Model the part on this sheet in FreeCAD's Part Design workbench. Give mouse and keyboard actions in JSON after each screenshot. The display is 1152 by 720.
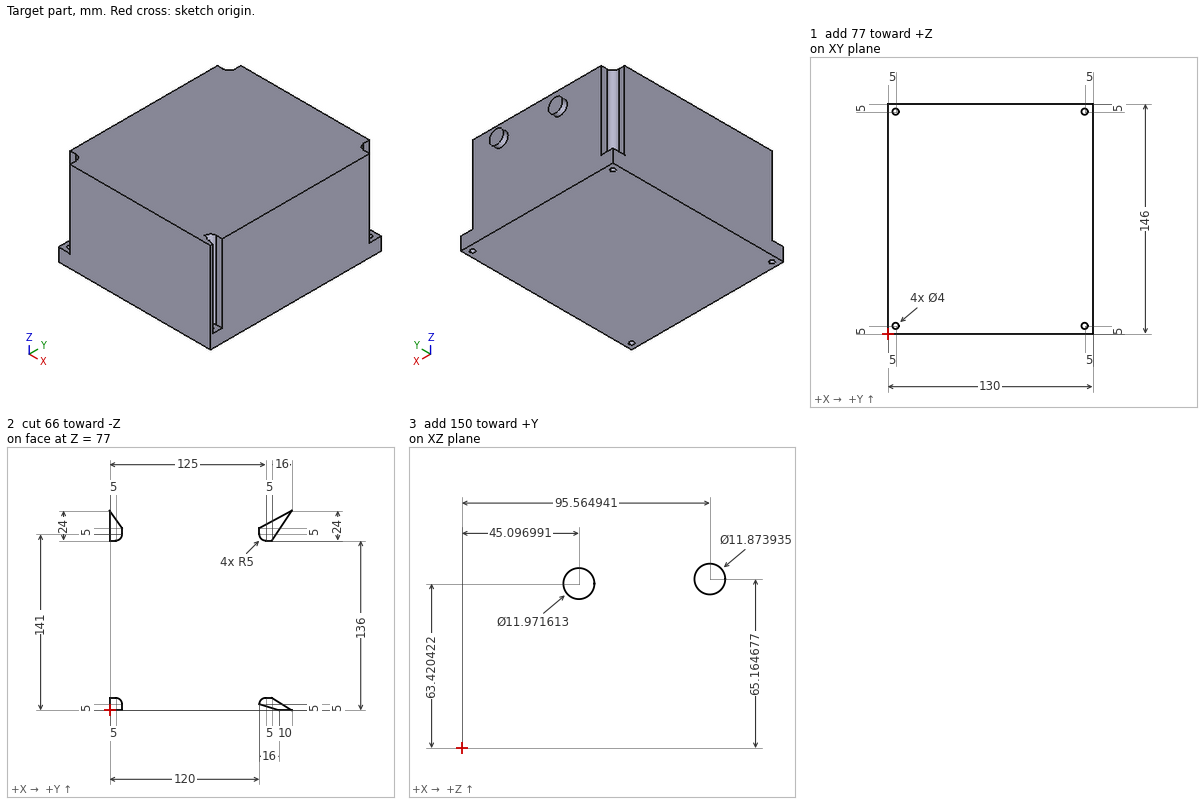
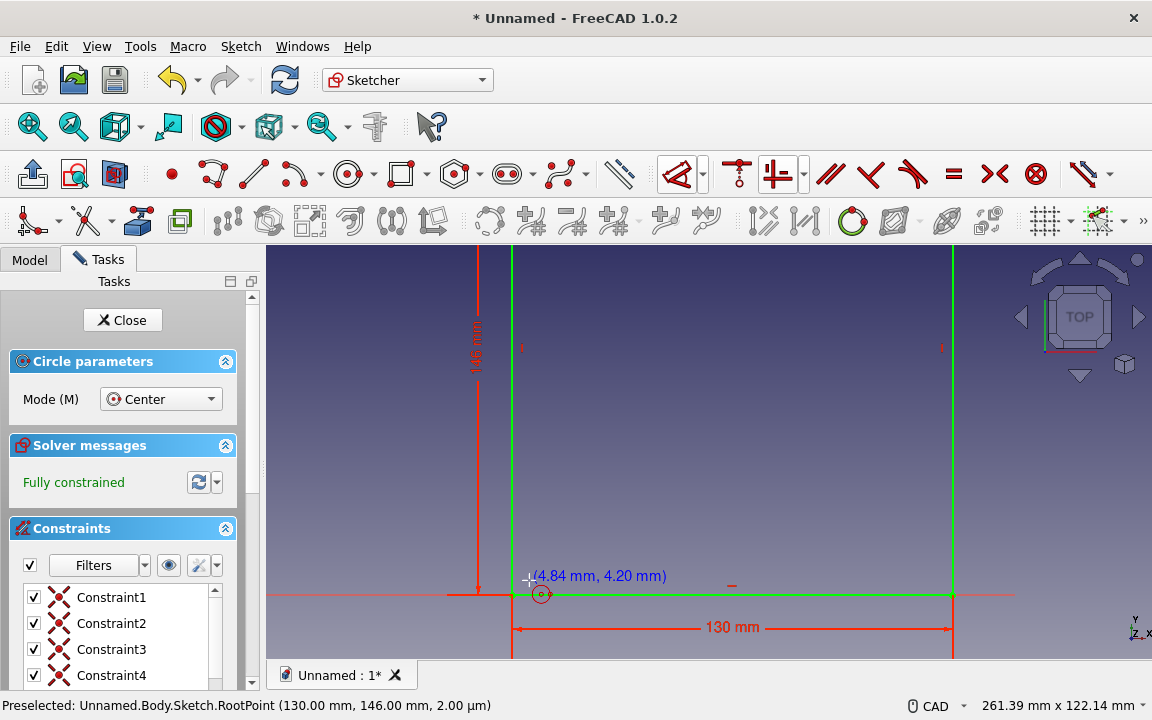
{"action": "left_click", "coordinate": [529, 578]}
{"action": "mouse_move", "coordinate": [534, 574]}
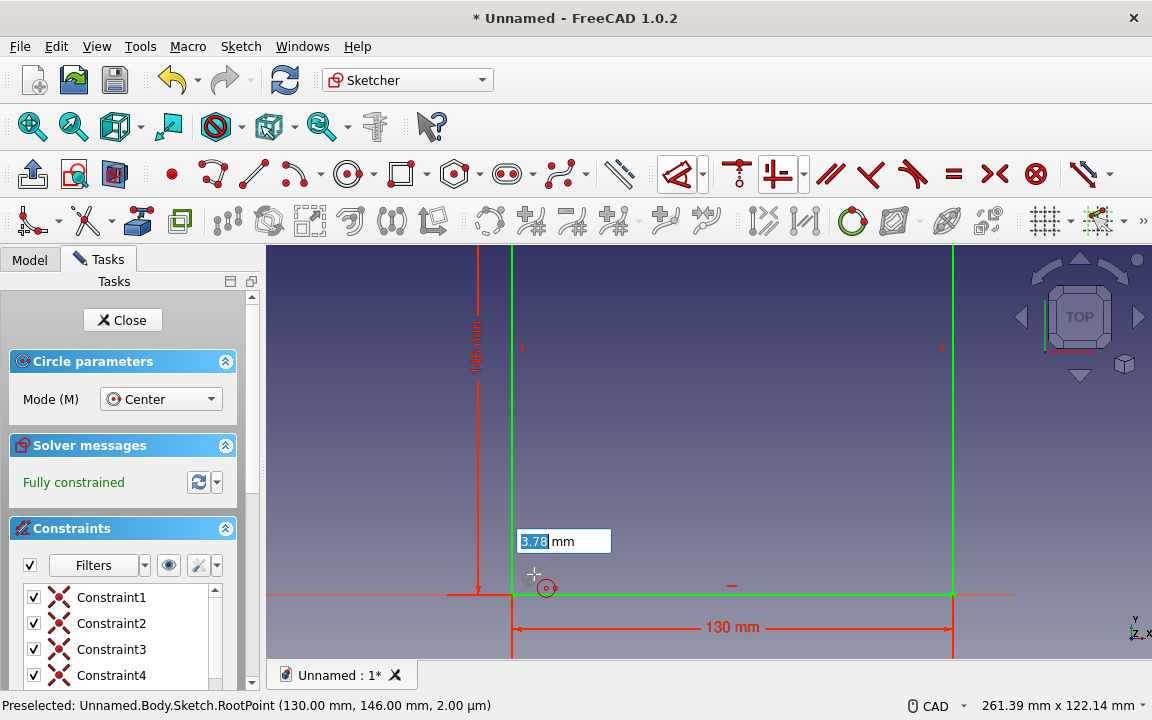
{"action": "type", "text": "4"}
{"action": "key", "text": "Return"}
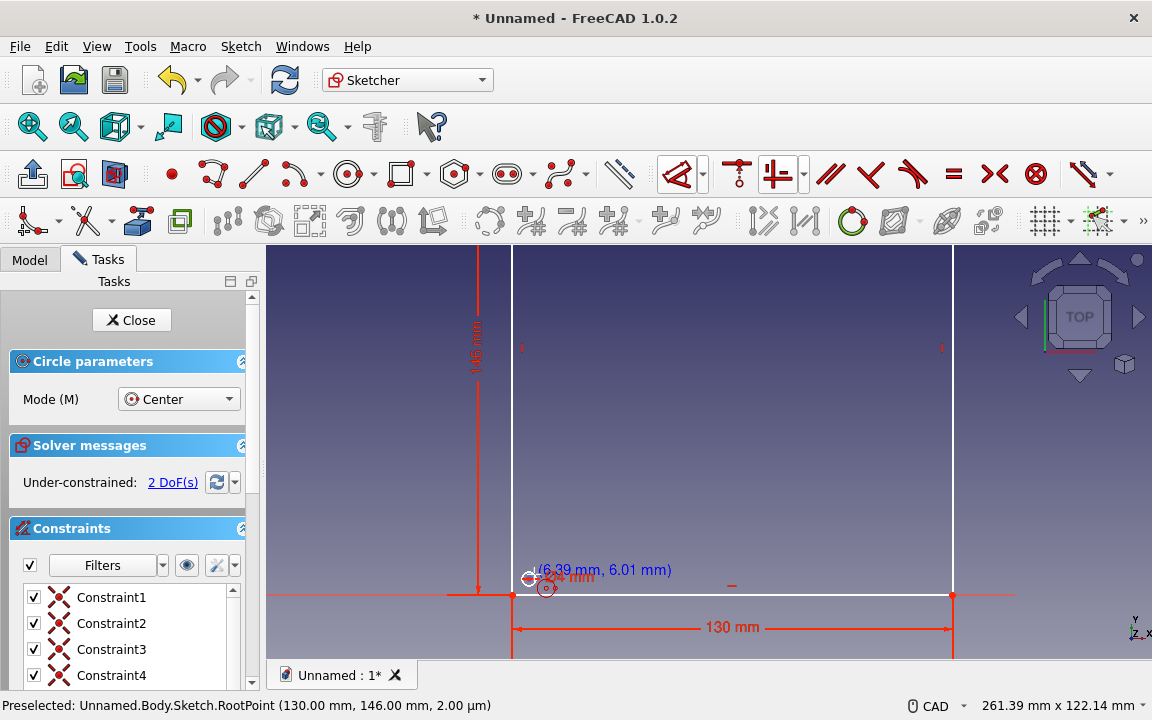
{"action": "scroll", "coordinate": [936, 578], "scroll_direction": "up", "scroll_amount": 7}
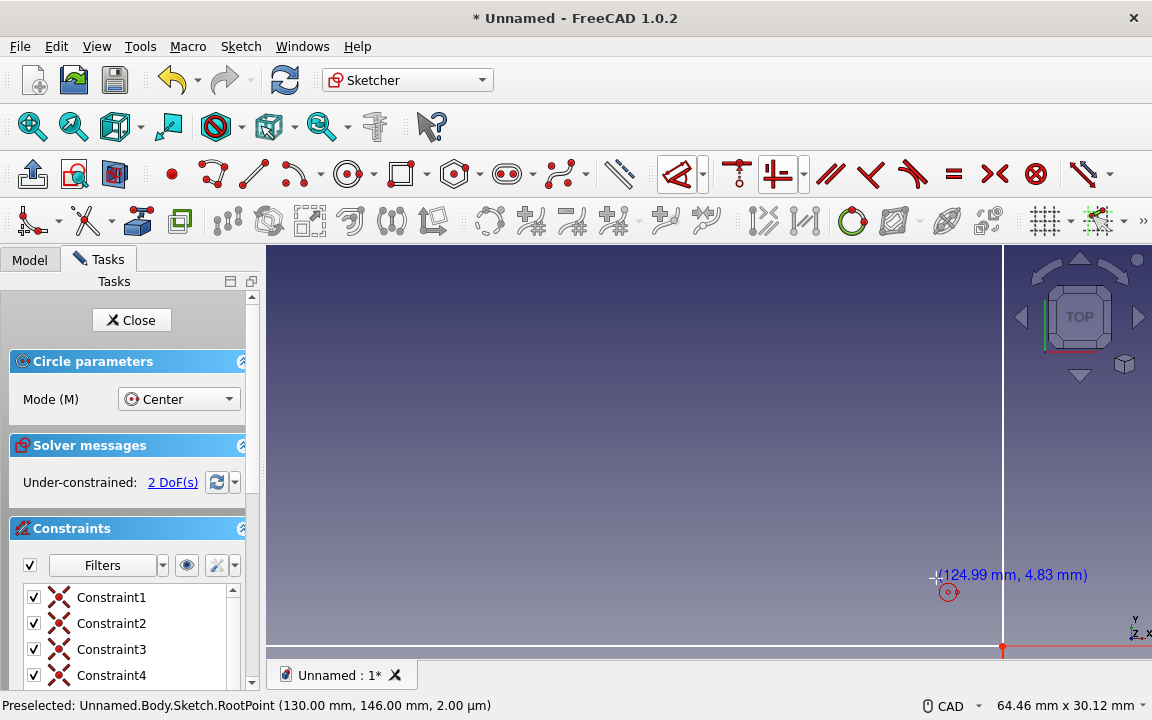
{"action": "scroll", "coordinate": [724, 579], "scroll_direction": "down", "scroll_amount": 10}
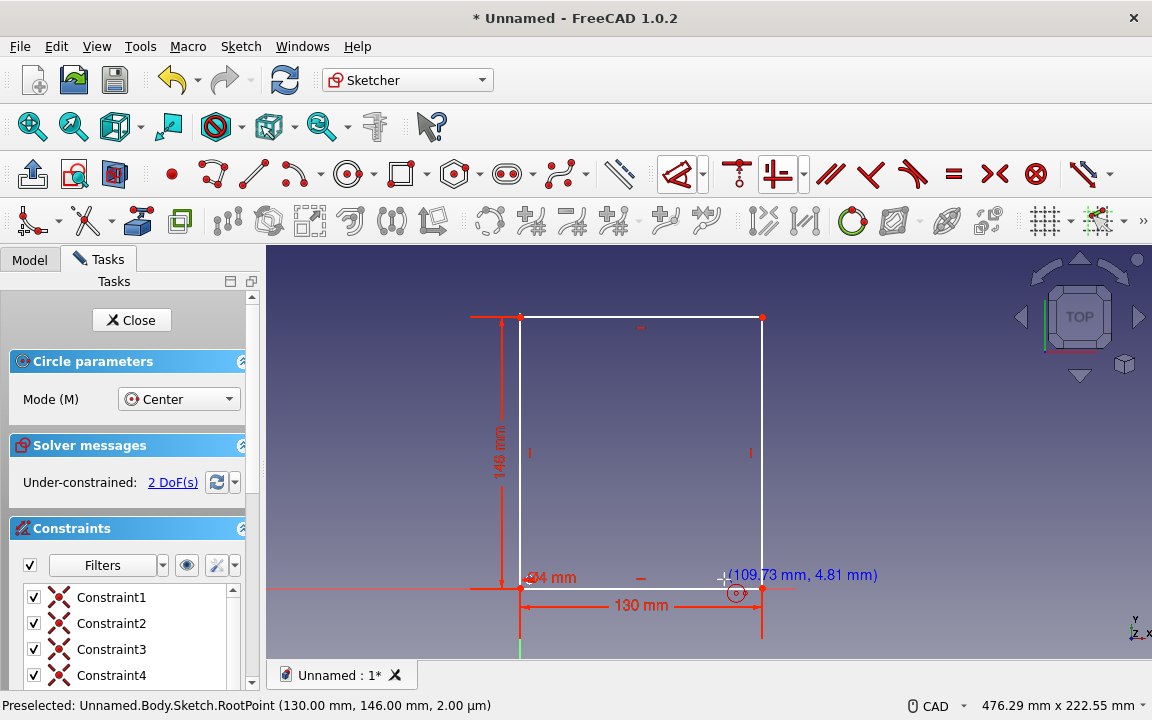
{"action": "scroll", "coordinate": [753, 579], "scroll_direction": "up", "scroll_amount": 3}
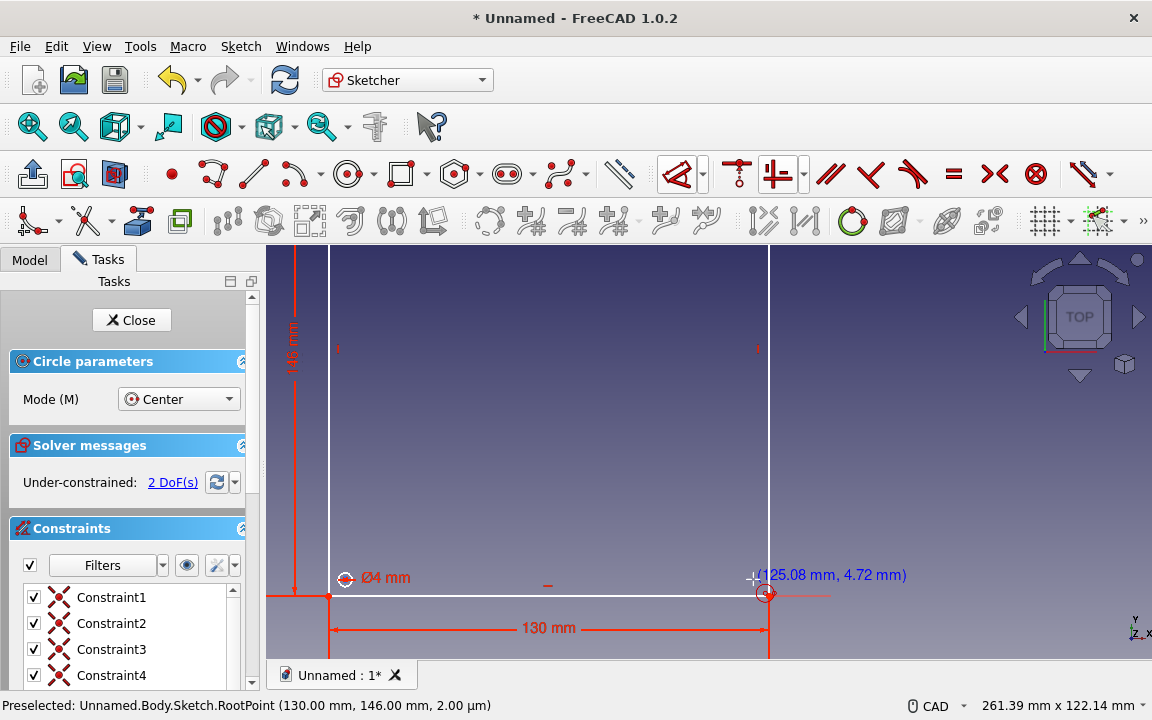
{"action": "left_click", "coordinate": [752, 579]}
{"action": "mouse_move", "coordinate": [747, 574]}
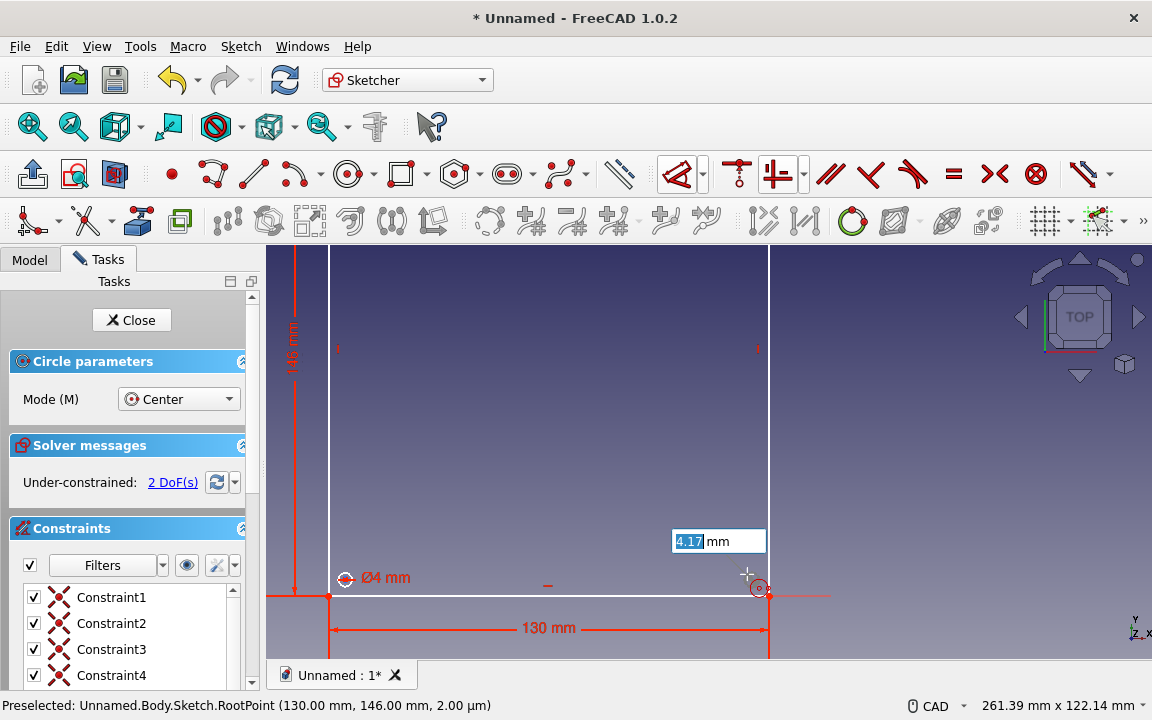
{"action": "type", "text": "4"}
{"action": "key", "text": "Return"}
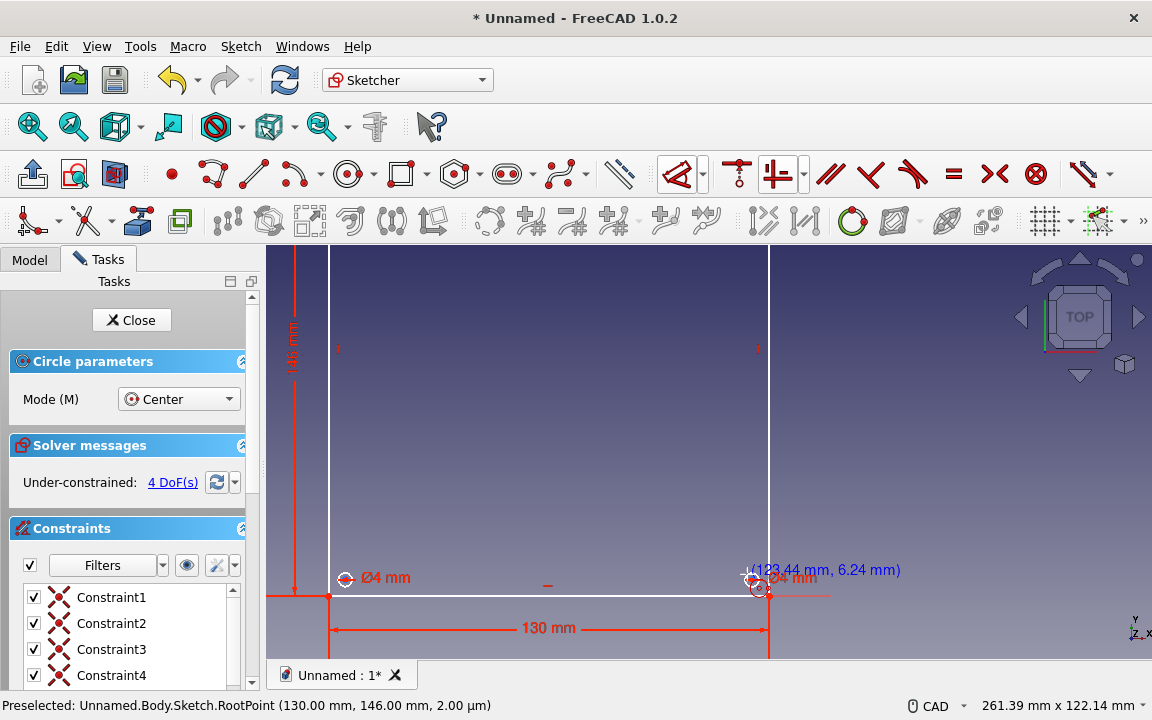
{"action": "scroll", "coordinate": [752, 578], "scroll_direction": "down", "scroll_amount": 3}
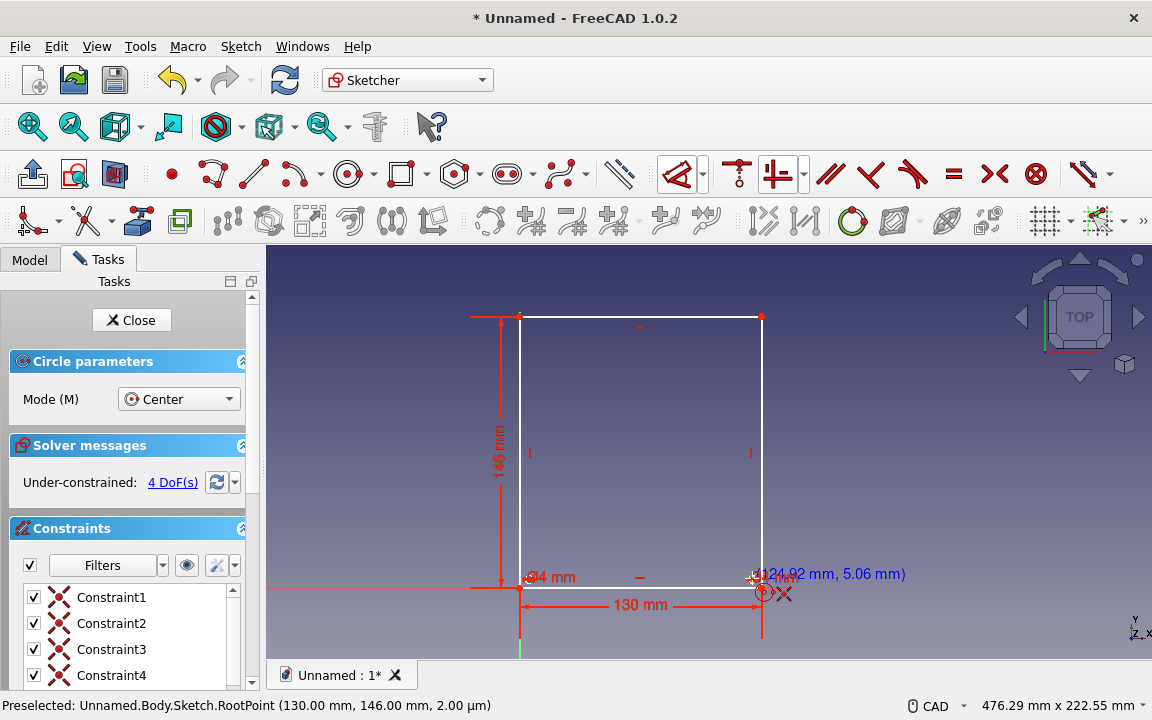
{"action": "scroll", "coordinate": [529, 326], "scroll_direction": "up", "scroll_amount": 10}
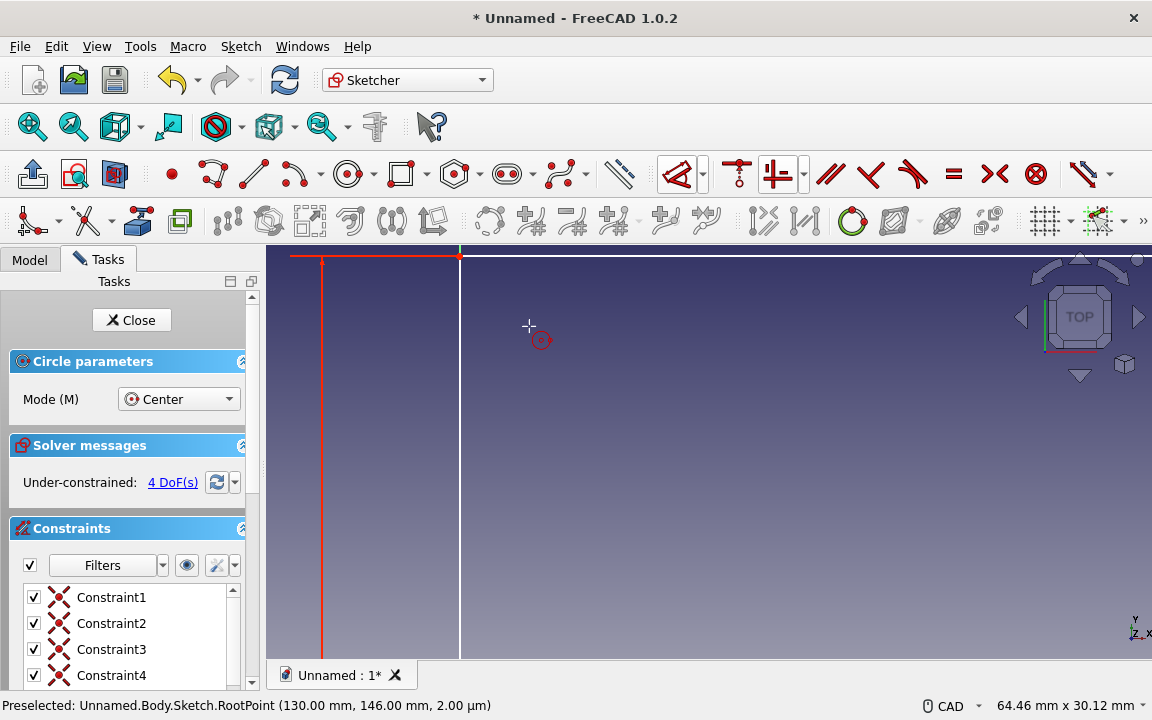
{"action": "scroll", "coordinate": [529, 326], "scroll_direction": "down", "scroll_amount": 10}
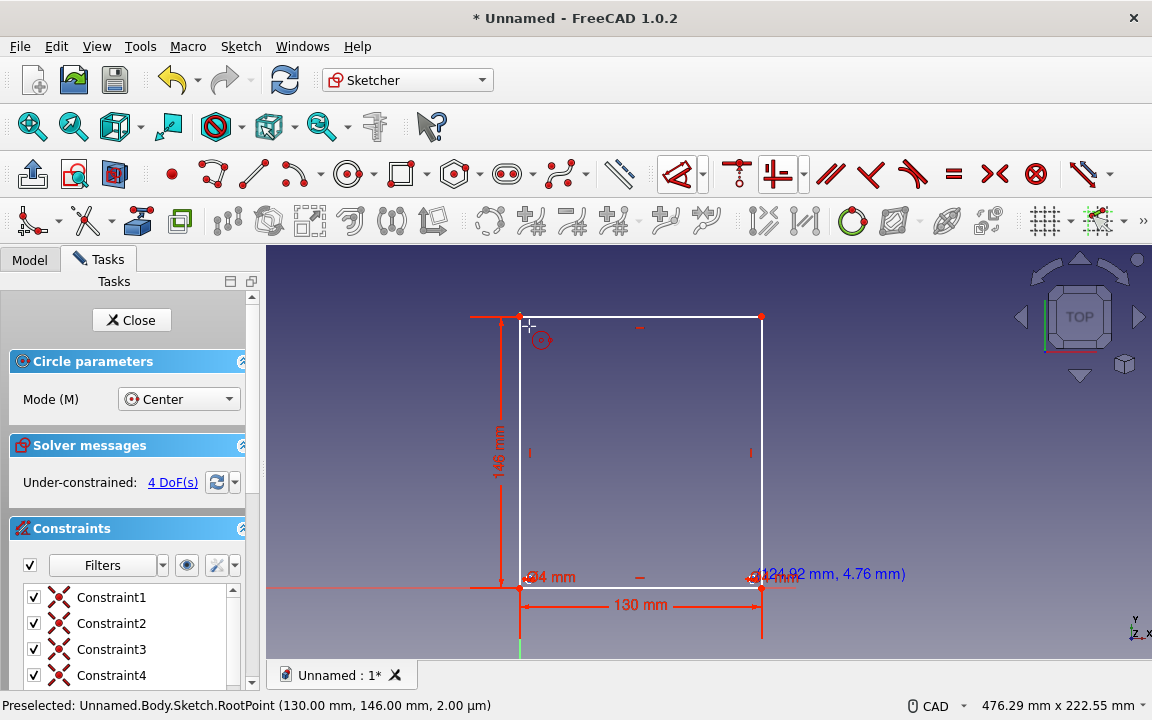
{"action": "scroll", "coordinate": [529, 326], "scroll_direction": "up", "scroll_amount": 3}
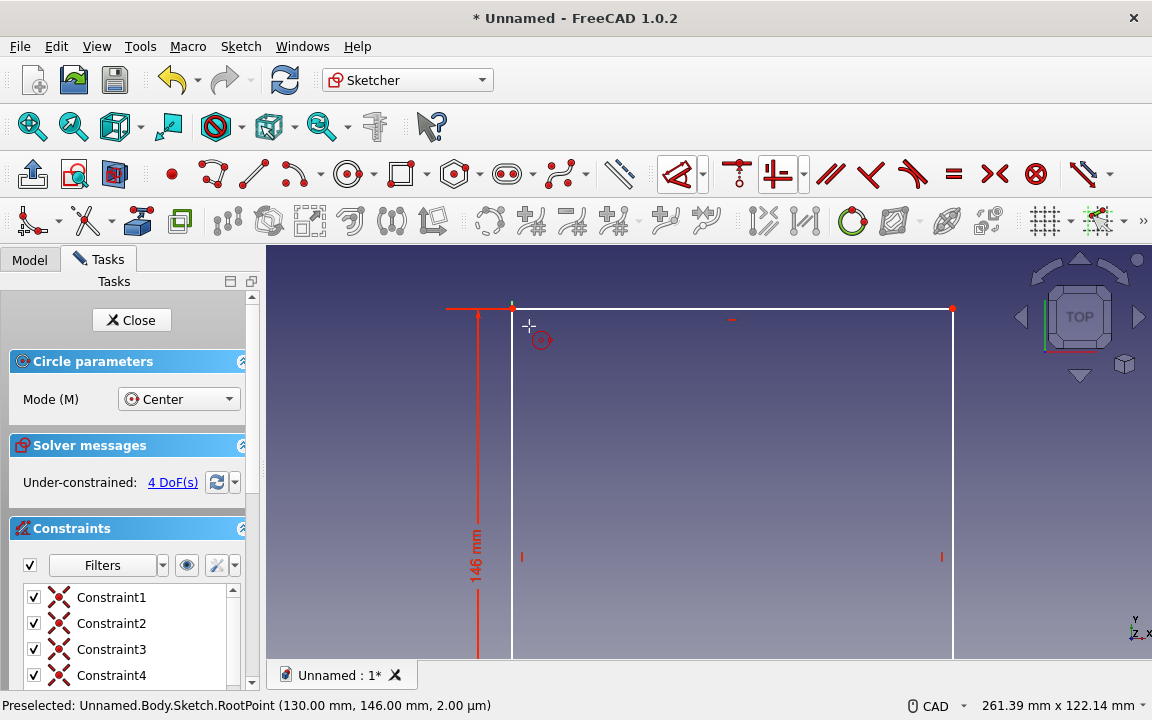
{"action": "left_click", "coordinate": [529, 326]}
{"action": "mouse_move", "coordinate": [534, 331]}